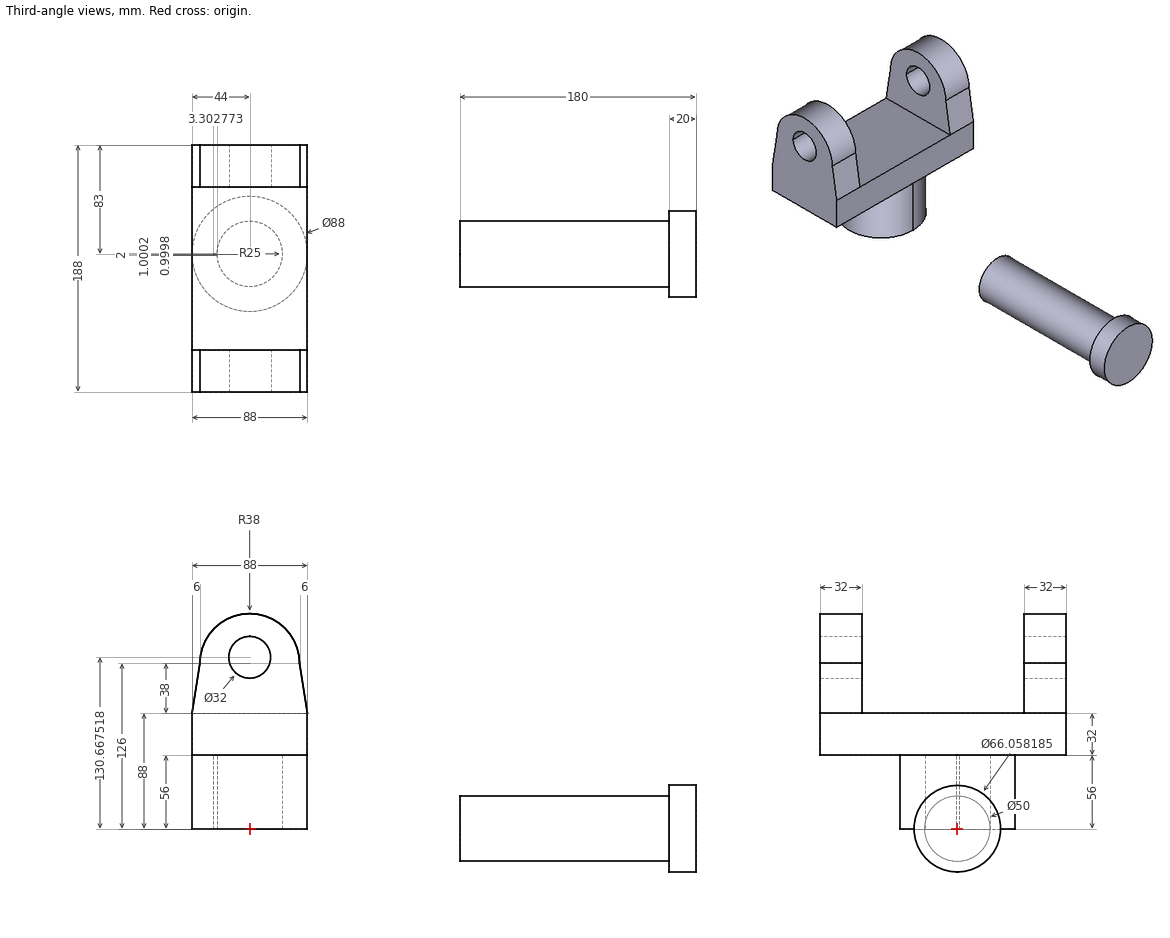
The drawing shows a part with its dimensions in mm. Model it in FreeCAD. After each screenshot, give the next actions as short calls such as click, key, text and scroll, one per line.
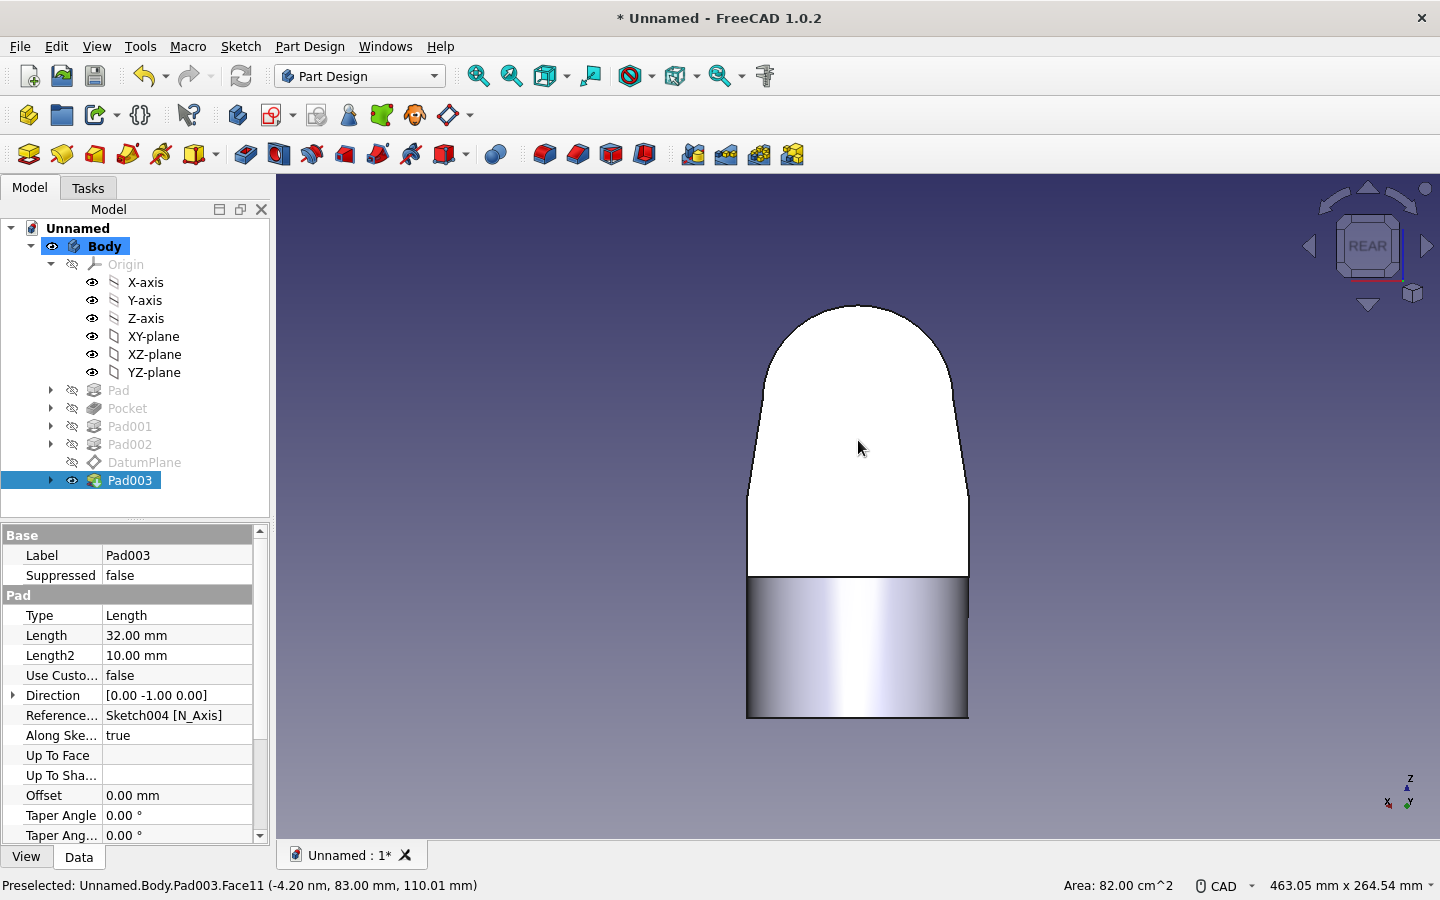
click(270, 116)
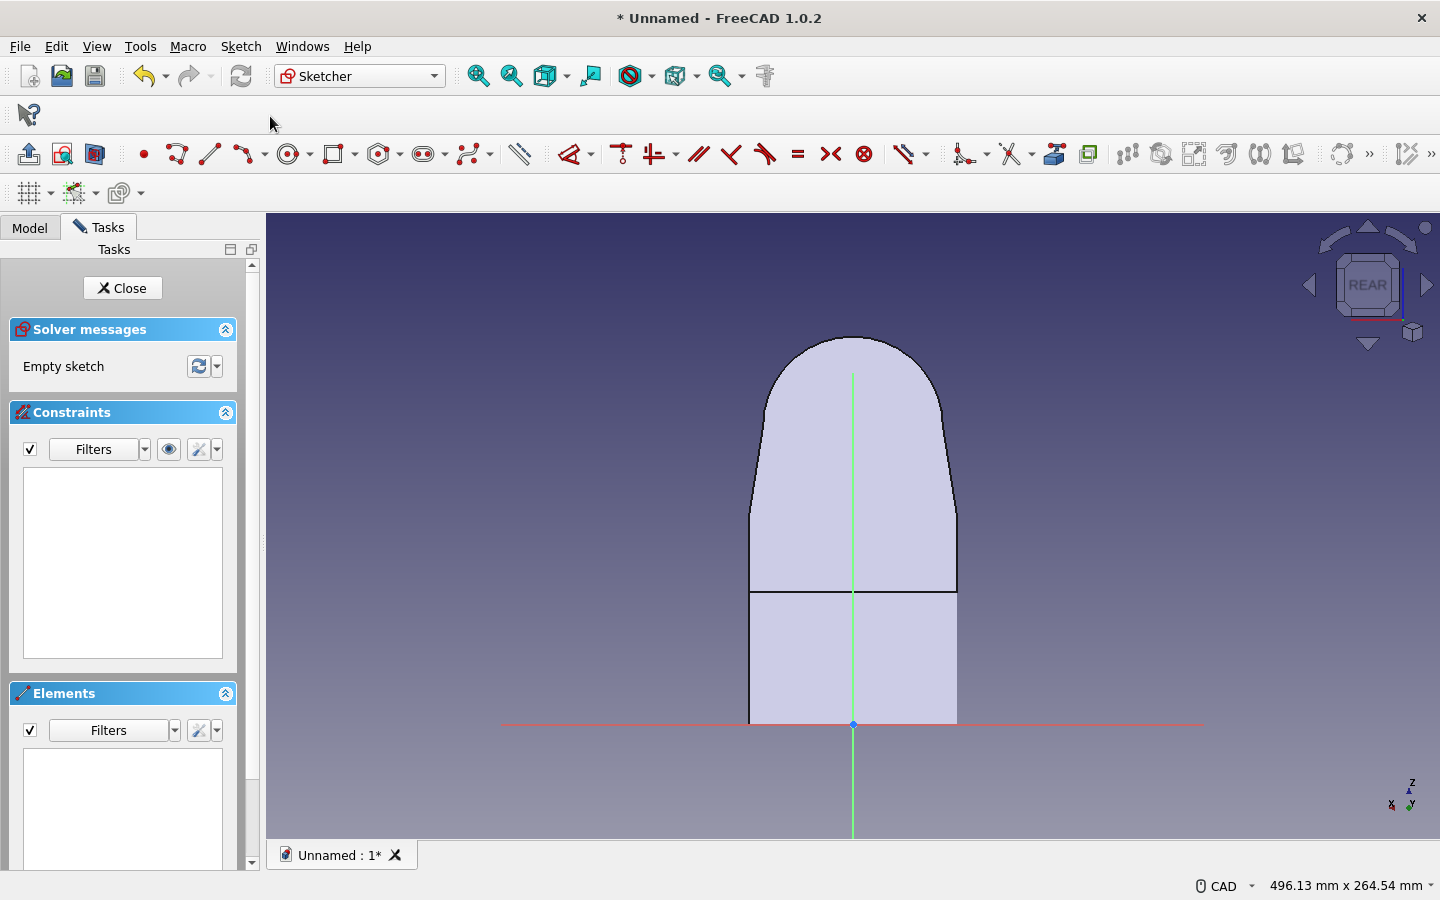
scroll(870, 388, up, 8)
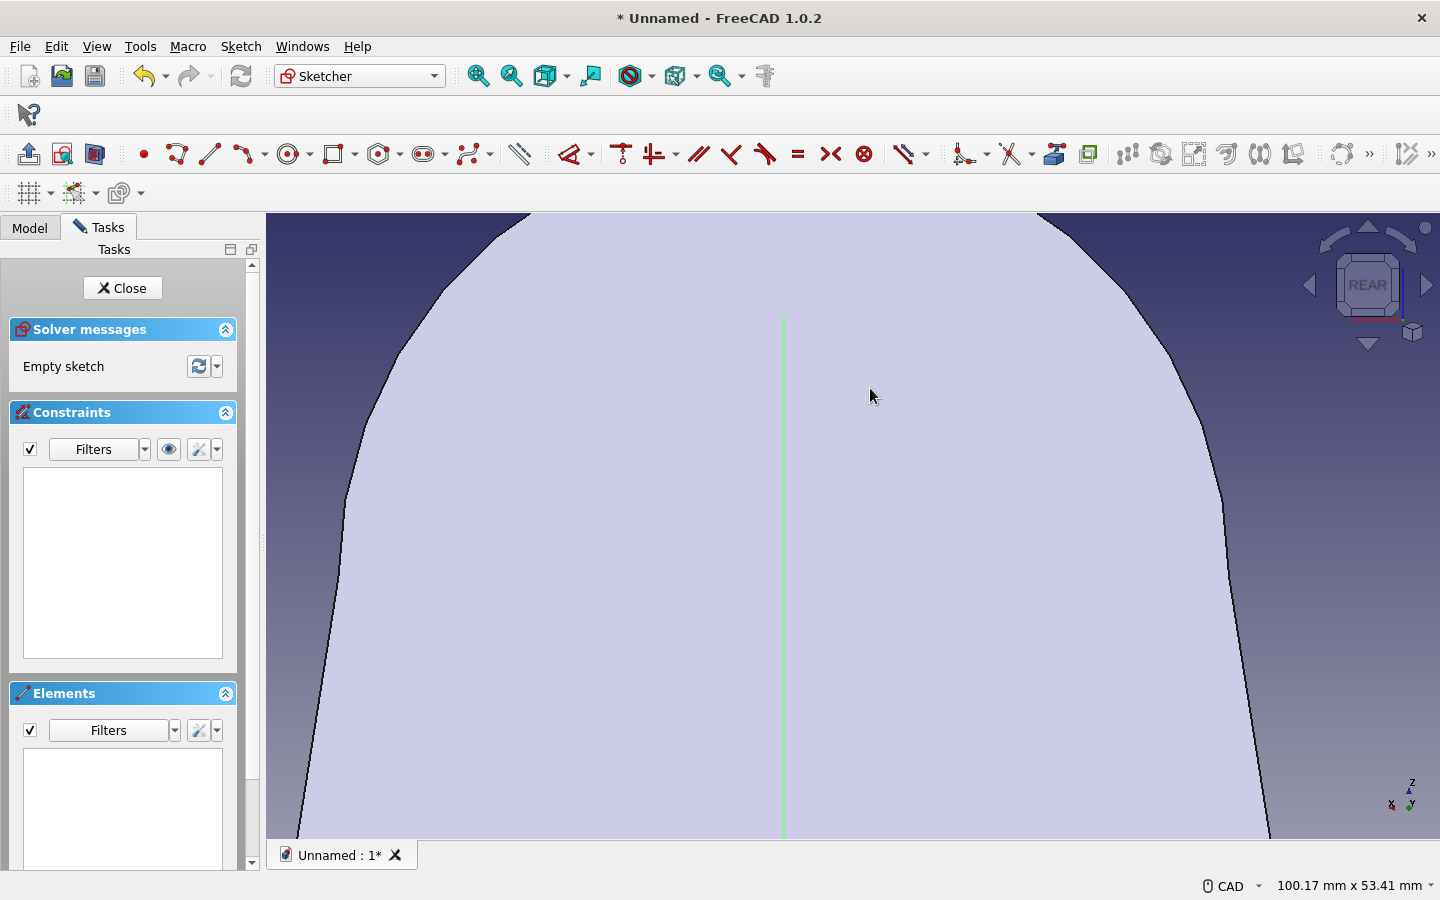
click(288, 154)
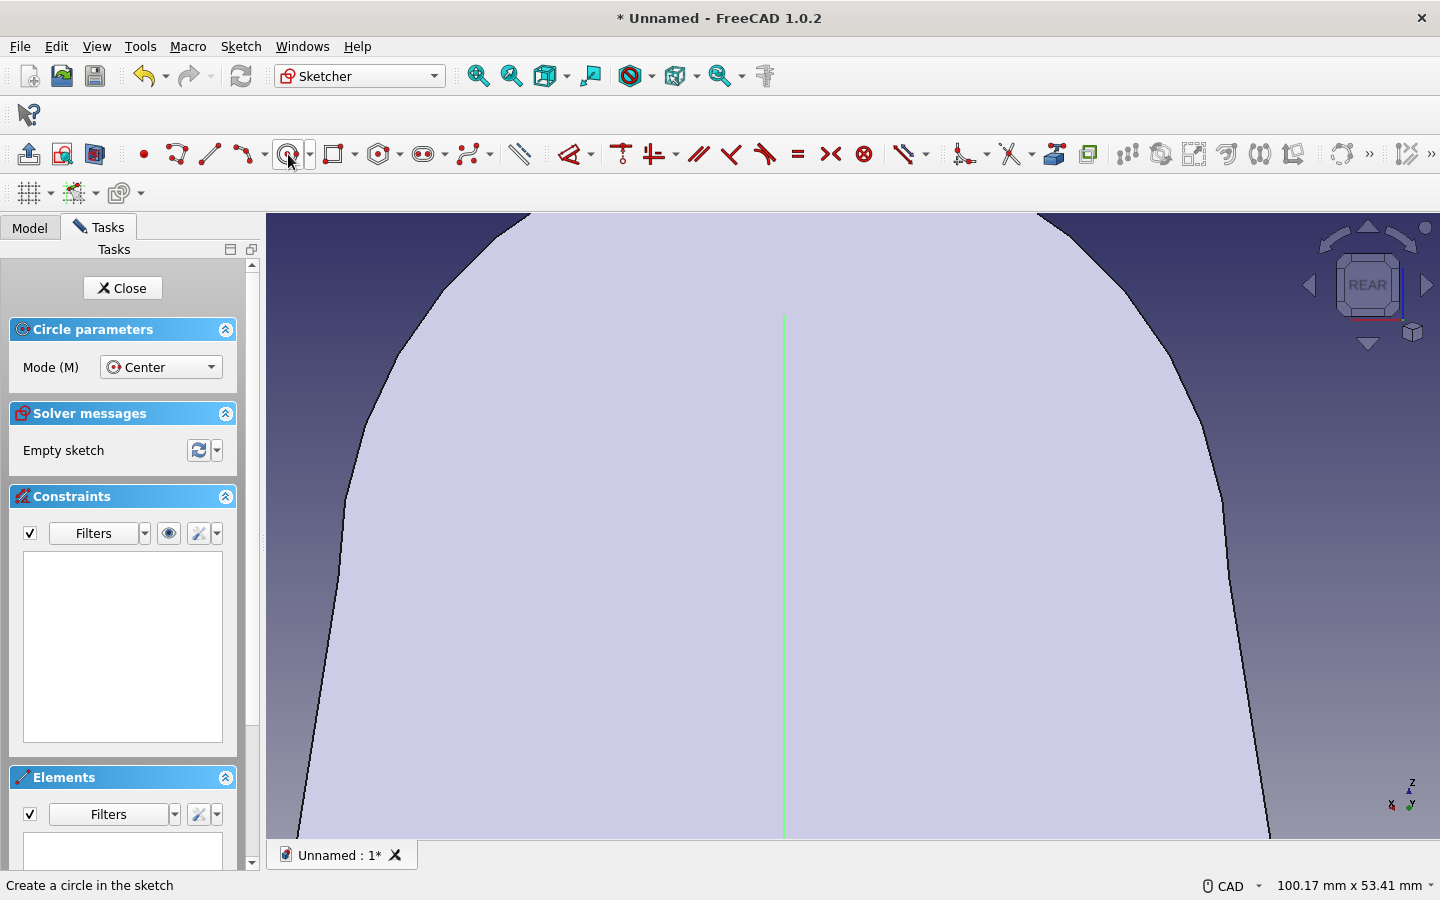
click(784, 523)
click(916, 390)
key(Escape)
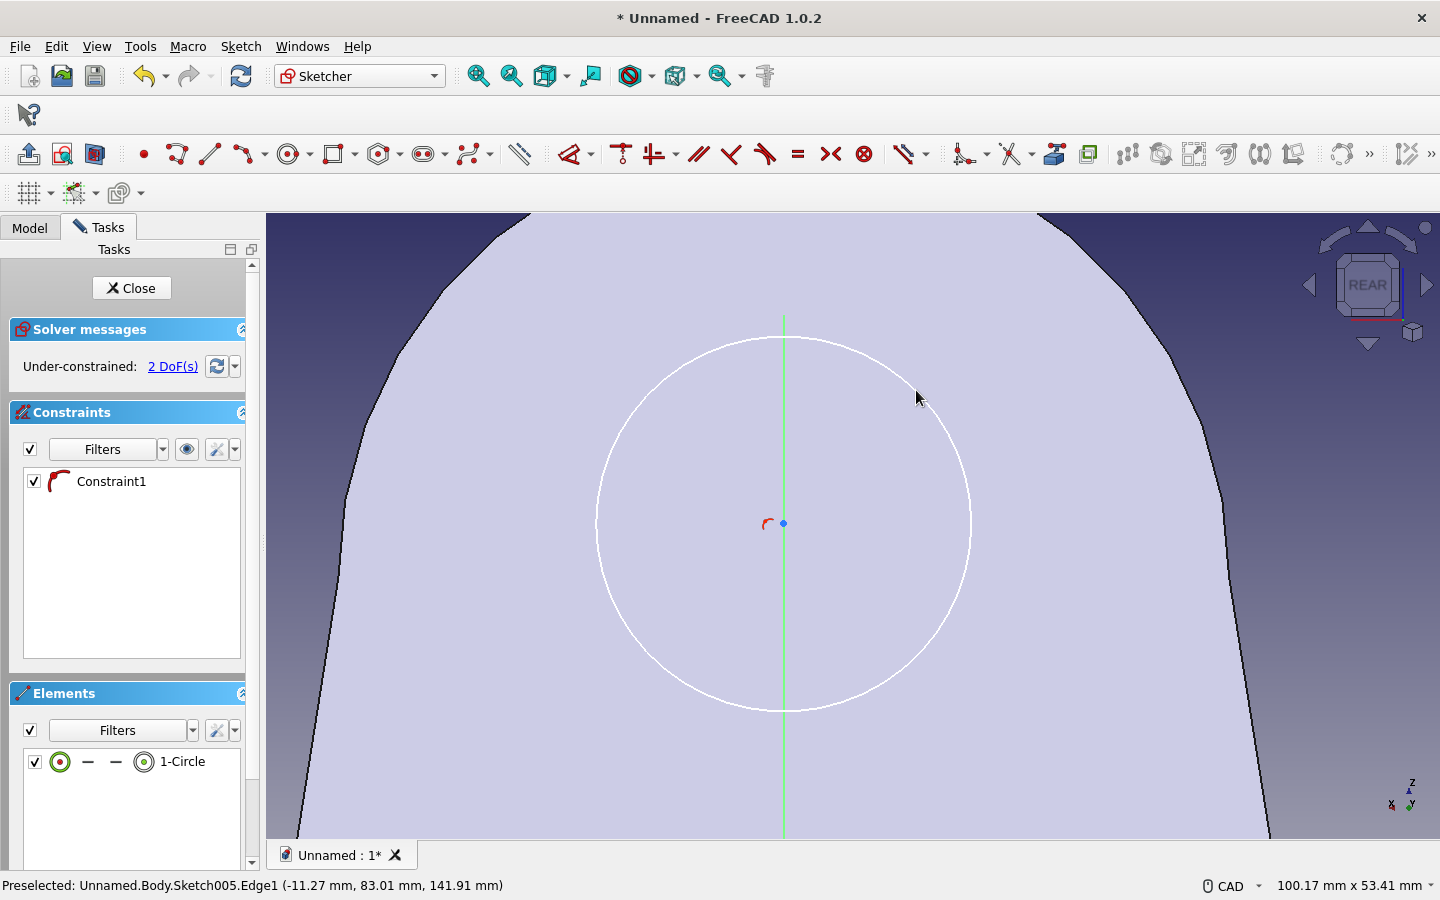
key(d)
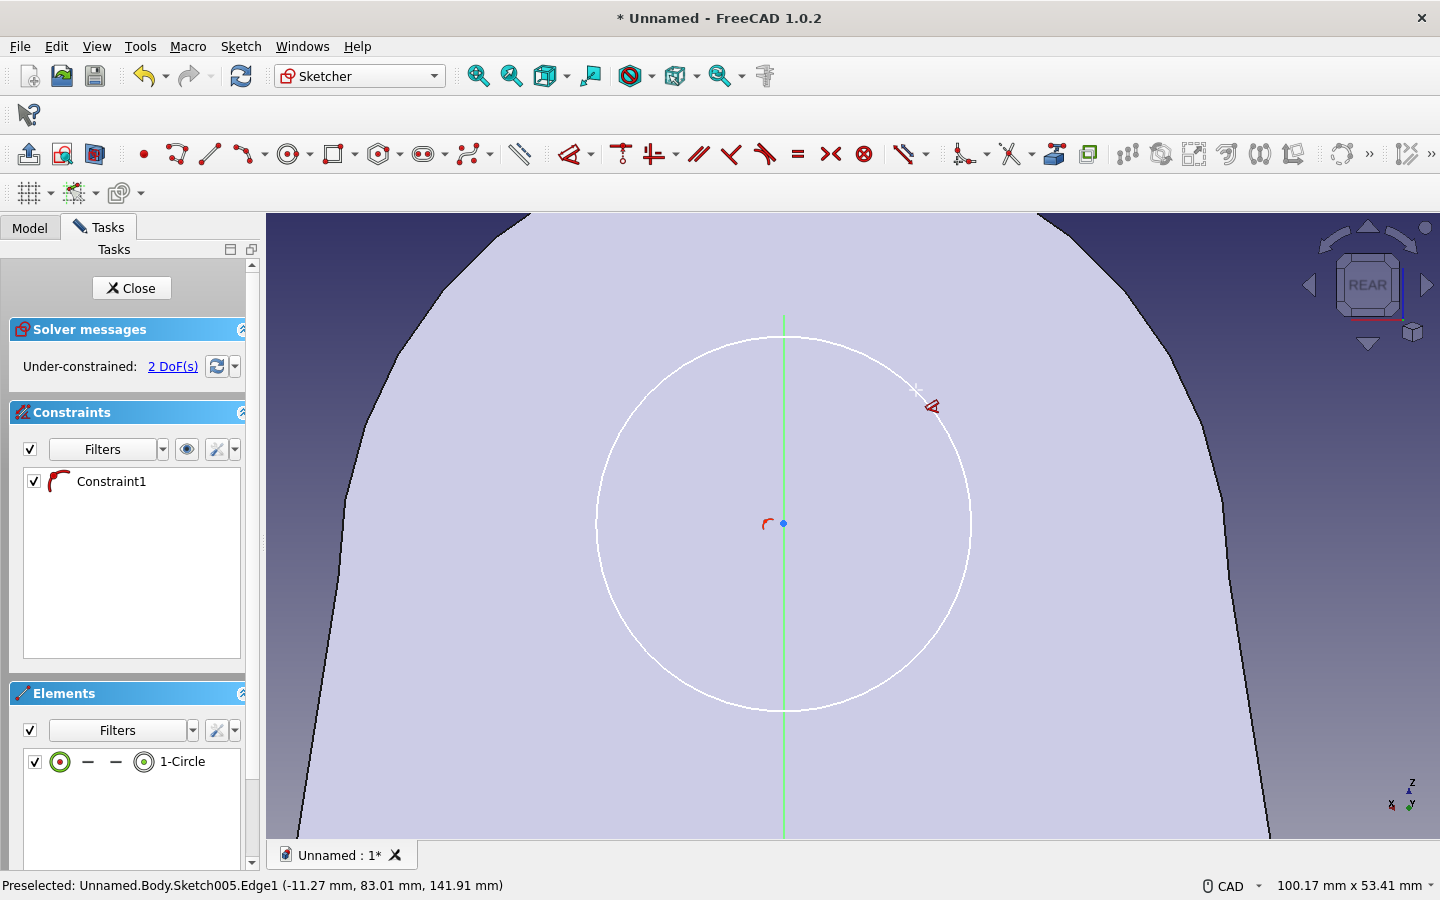
click(916, 391)
click(939, 368)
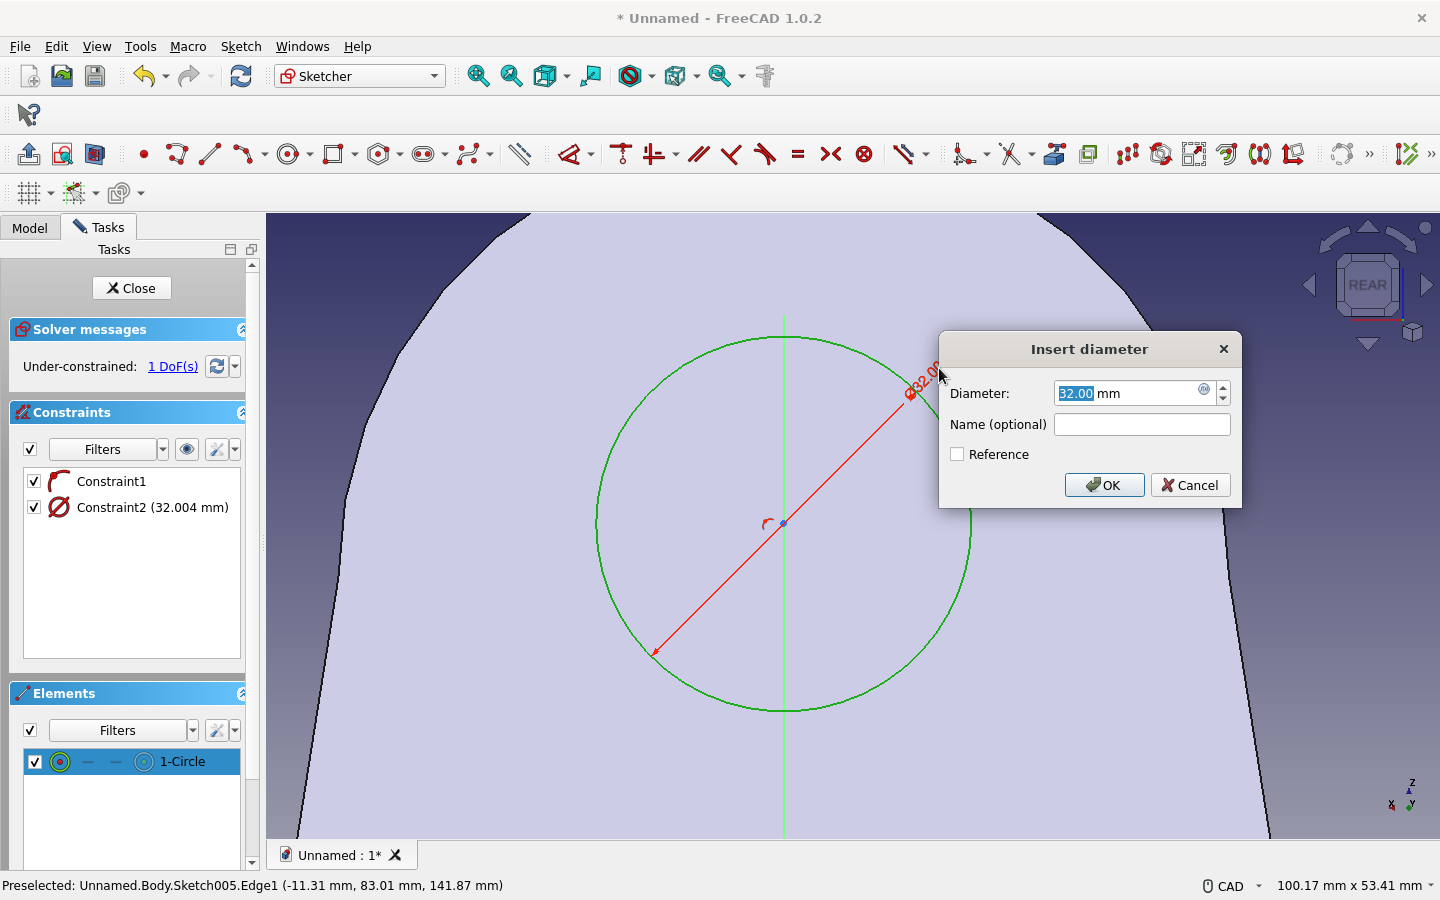
text(32)
key(Return)